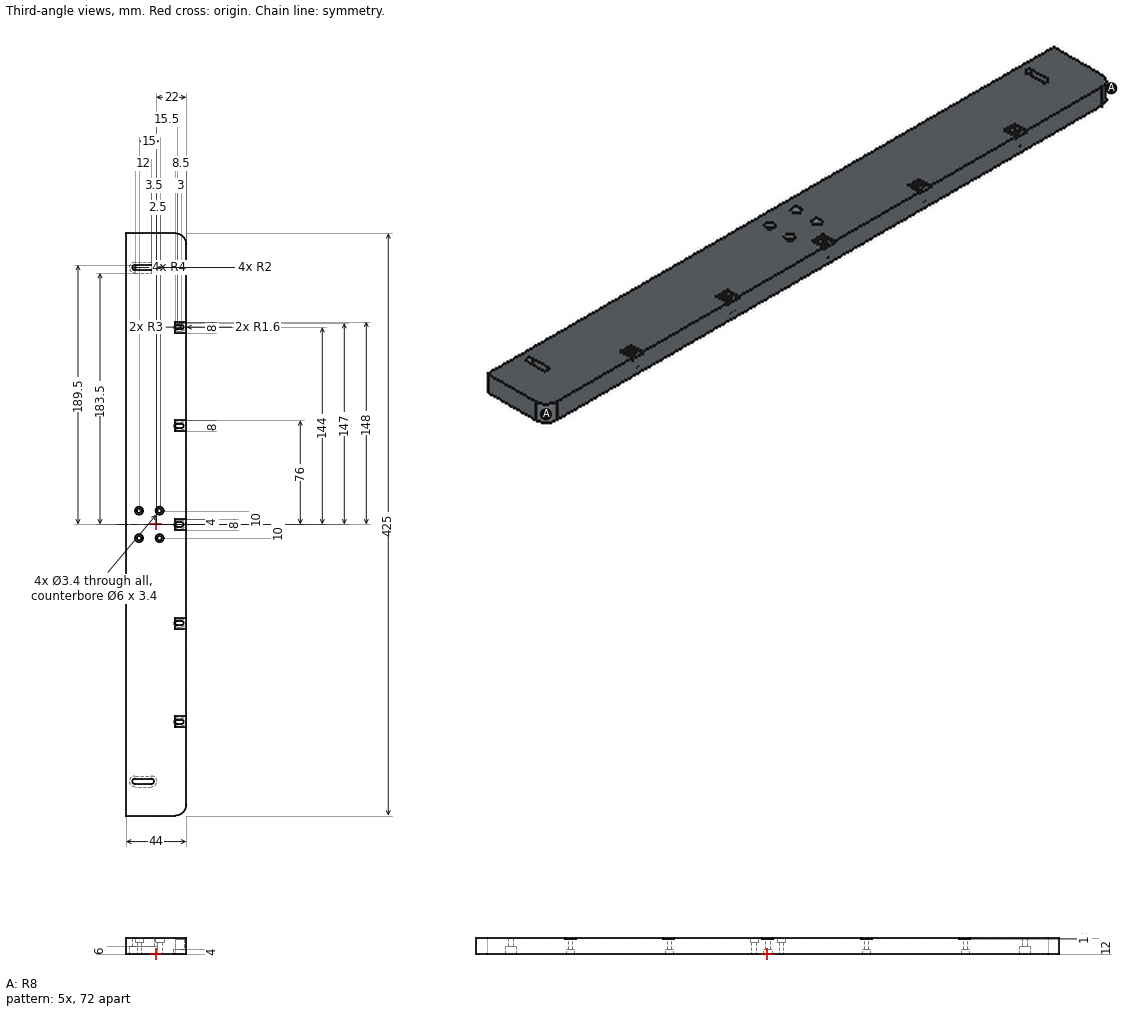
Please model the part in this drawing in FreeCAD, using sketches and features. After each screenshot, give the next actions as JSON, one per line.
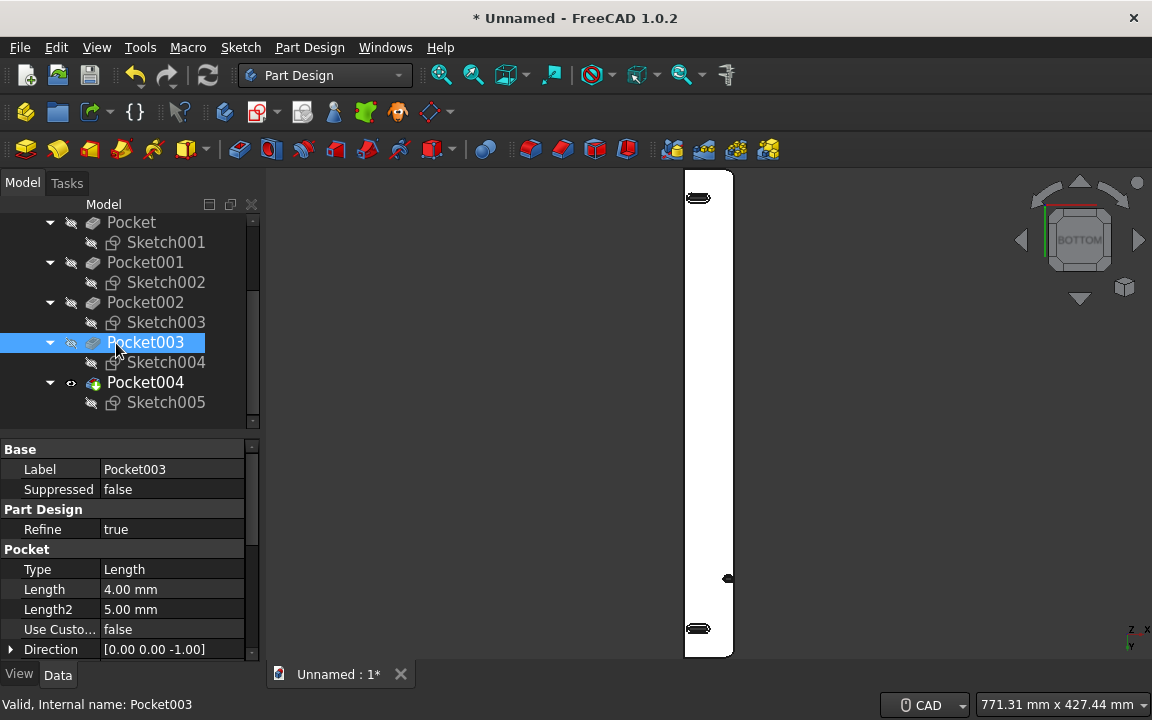
{"action": "left_click", "coordinate": [116, 383], "text": "ctrl"}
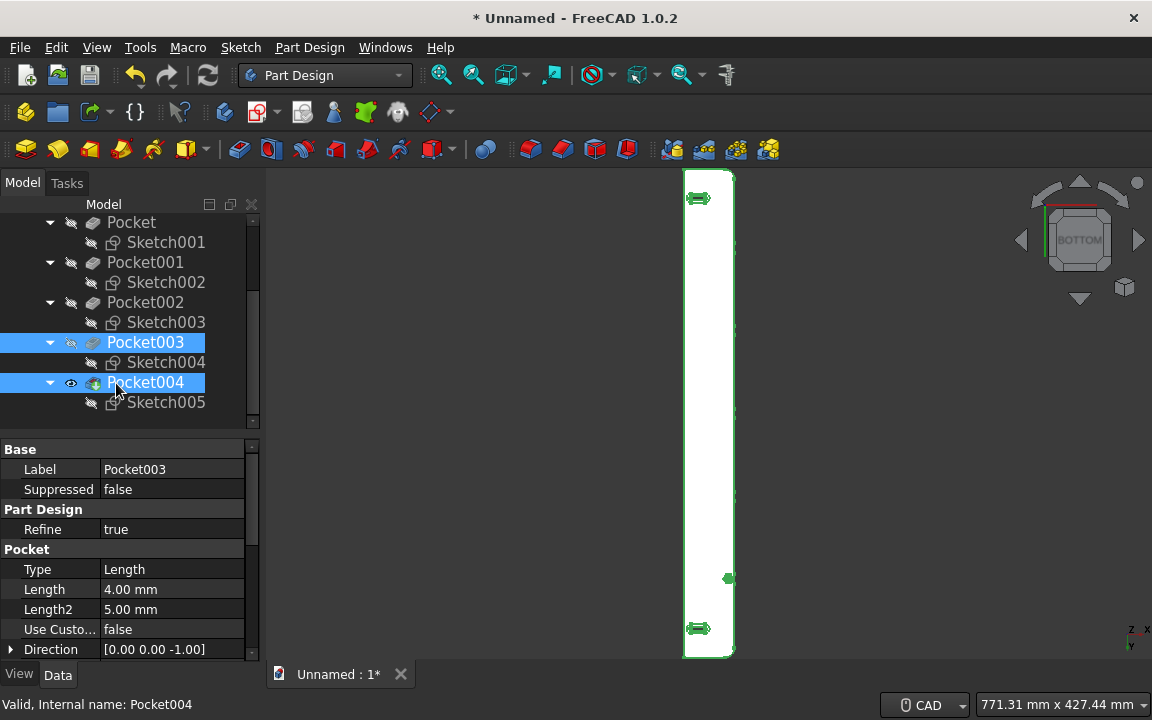
{"action": "left_click", "coordinate": [704, 150]}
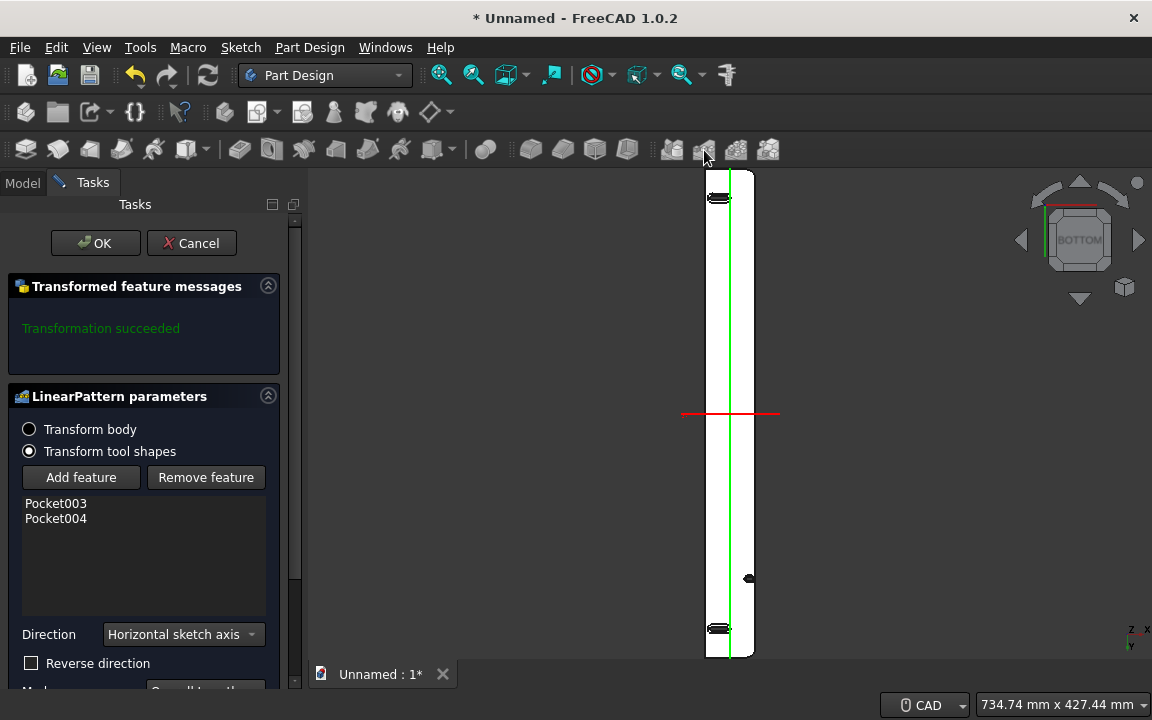
{"action": "left_click", "coordinate": [184, 634]}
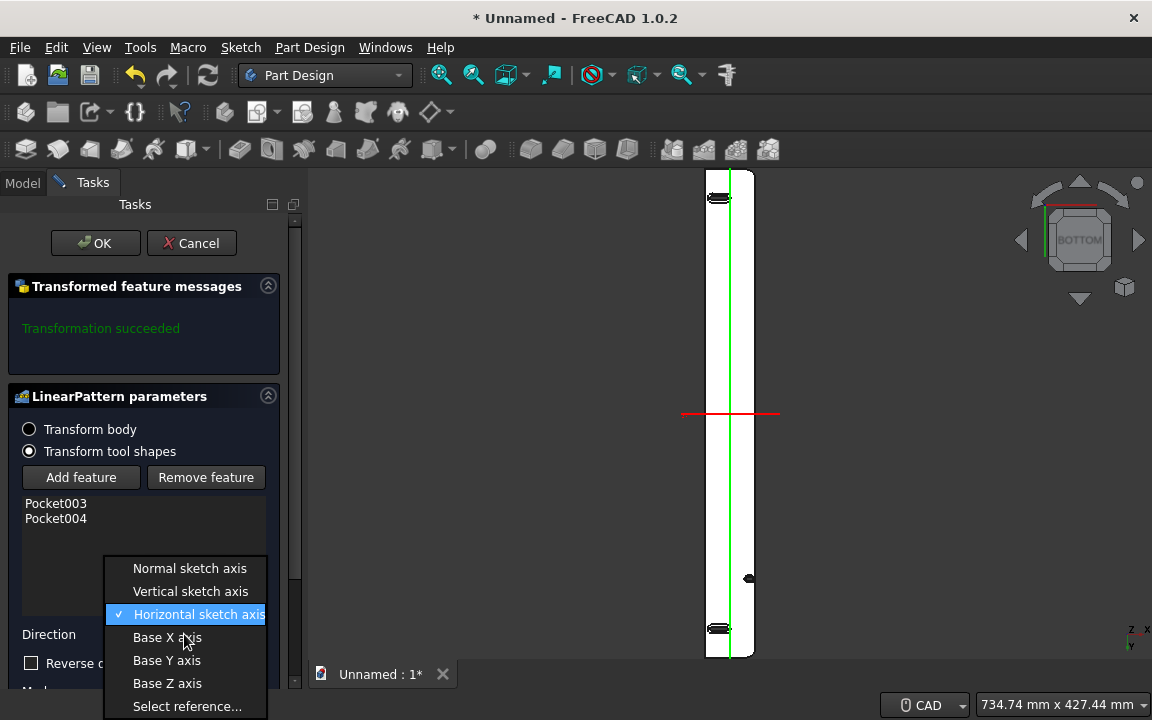
{"action": "left_click", "coordinate": [184, 660]}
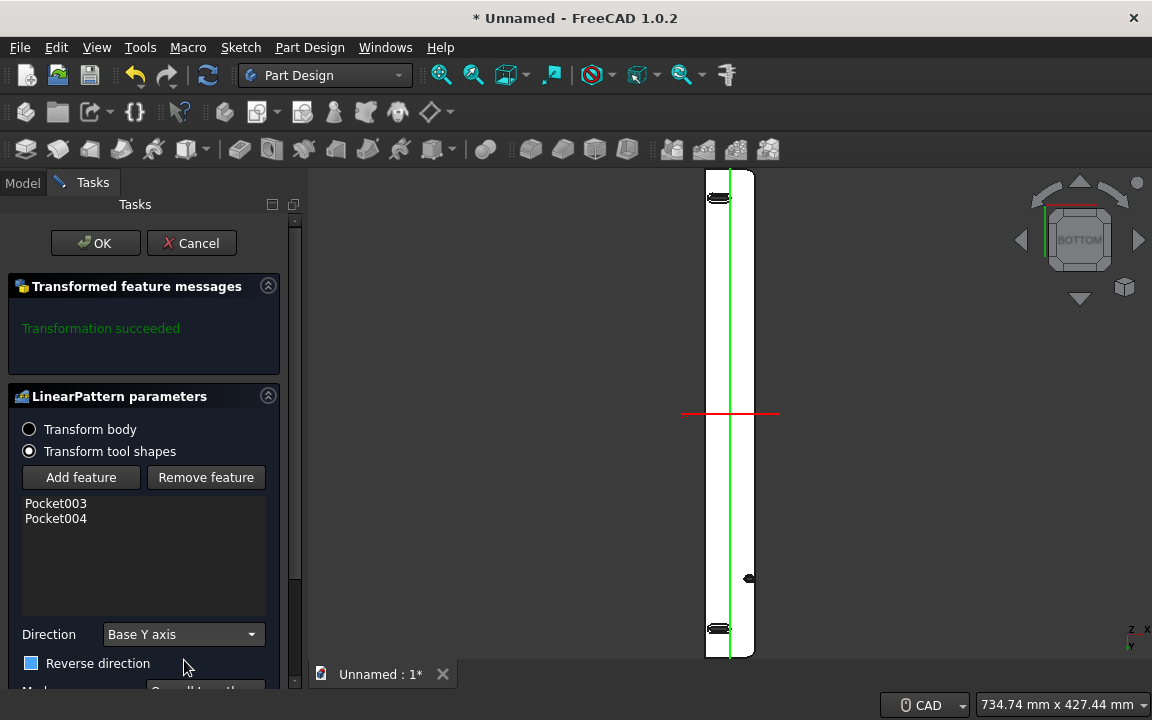
{"action": "scroll", "coordinate": [295, 451], "scroll_direction": "down", "scroll_amount": 2}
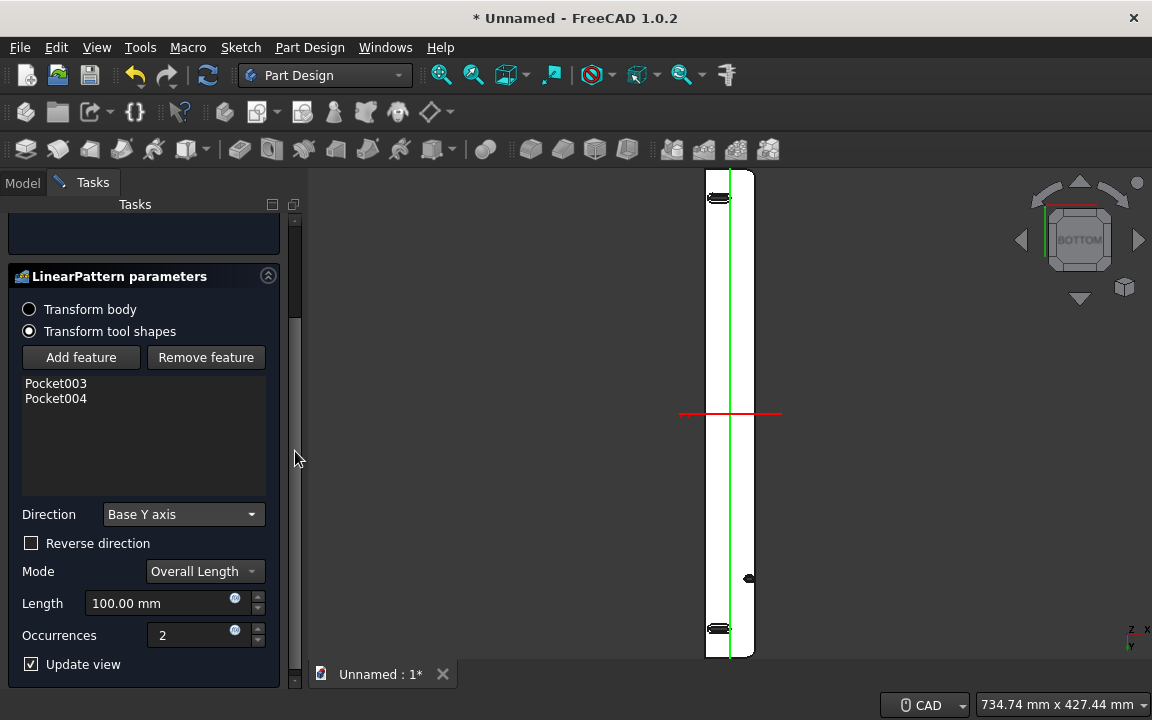
{"action": "left_click", "coordinate": [206, 572]}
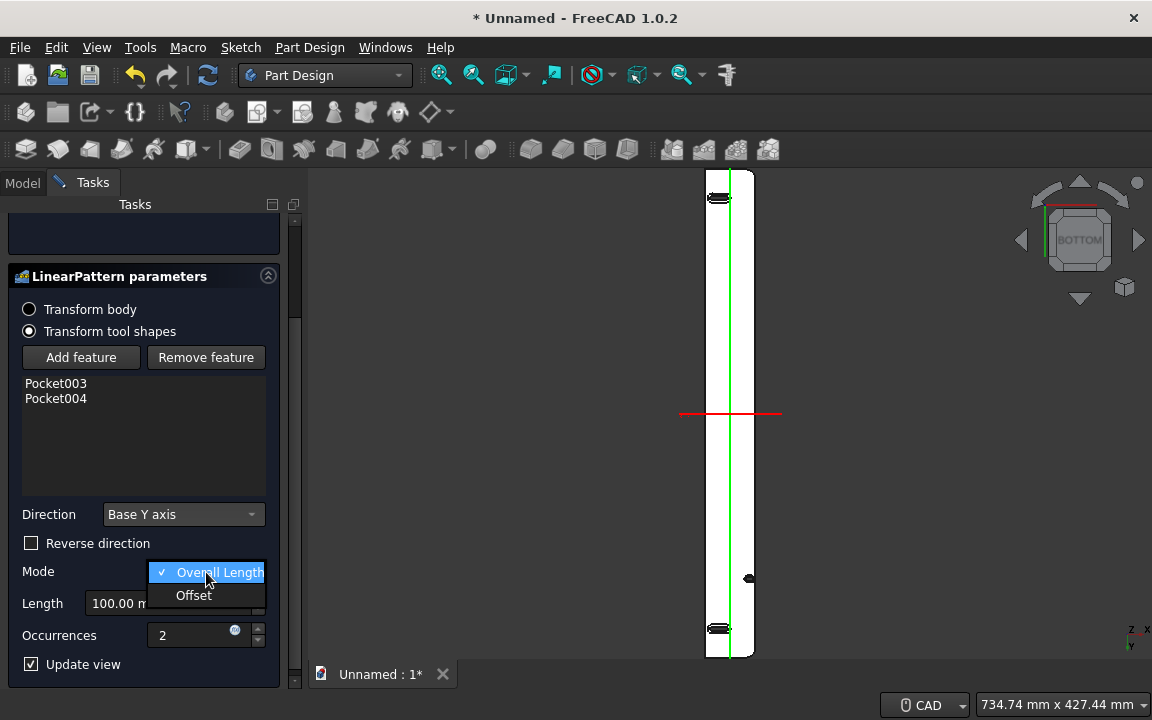
{"action": "left_click", "coordinate": [206, 596]}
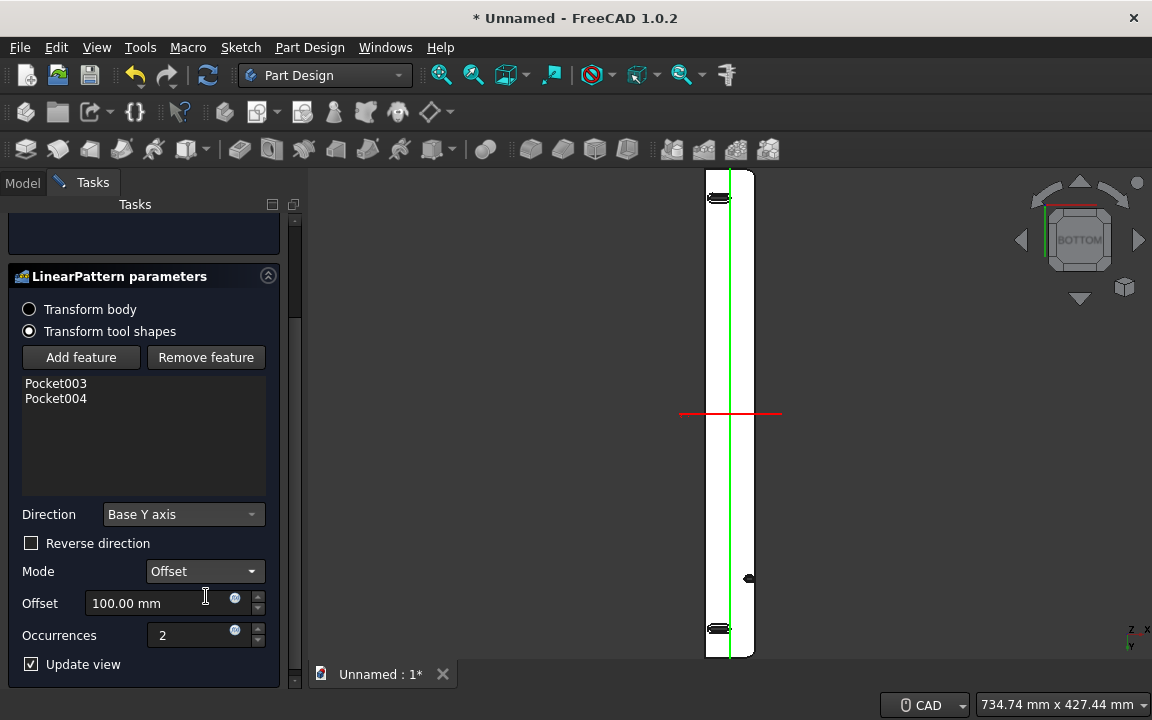
{"action": "triple_click", "coordinate": [168, 603]}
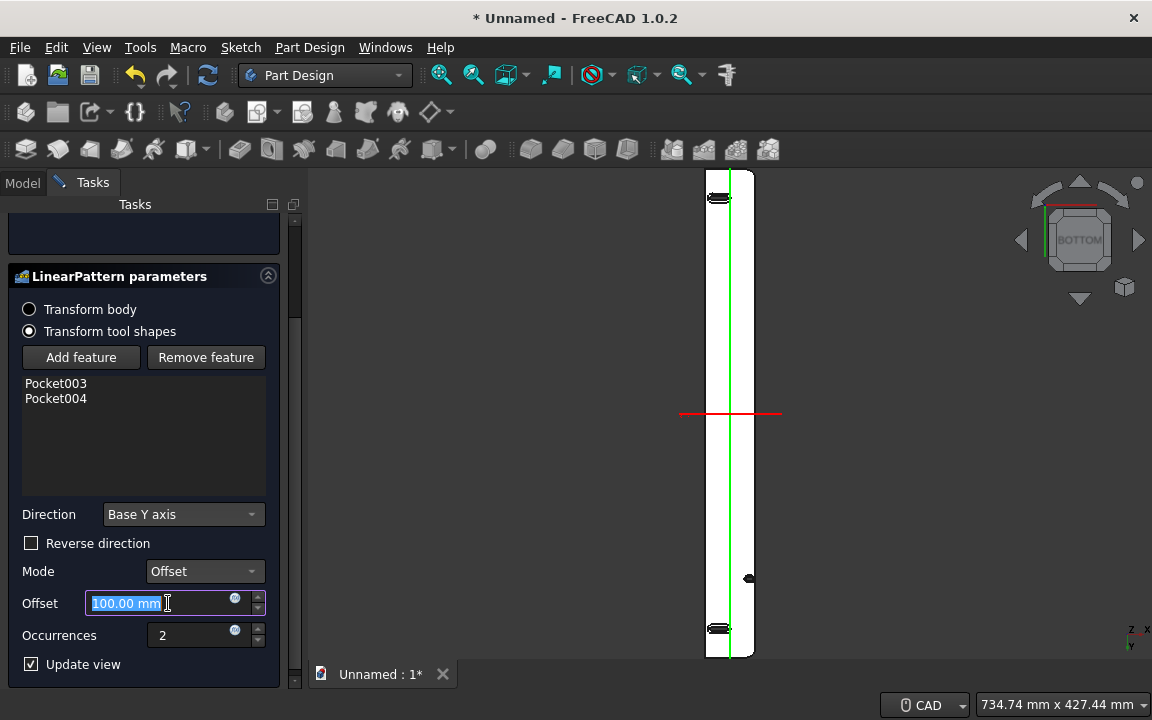
{"action": "type", "text": "72"}
{"action": "key", "text": "Tab"}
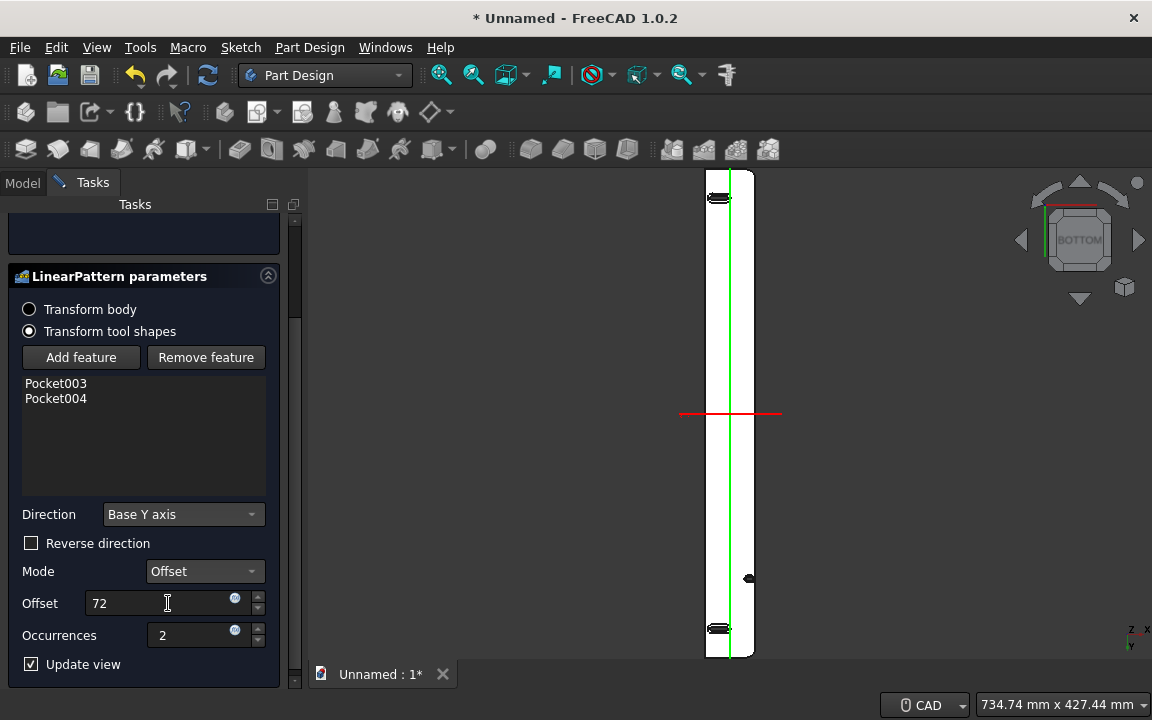
{"action": "triple_click", "coordinate": [198, 635]}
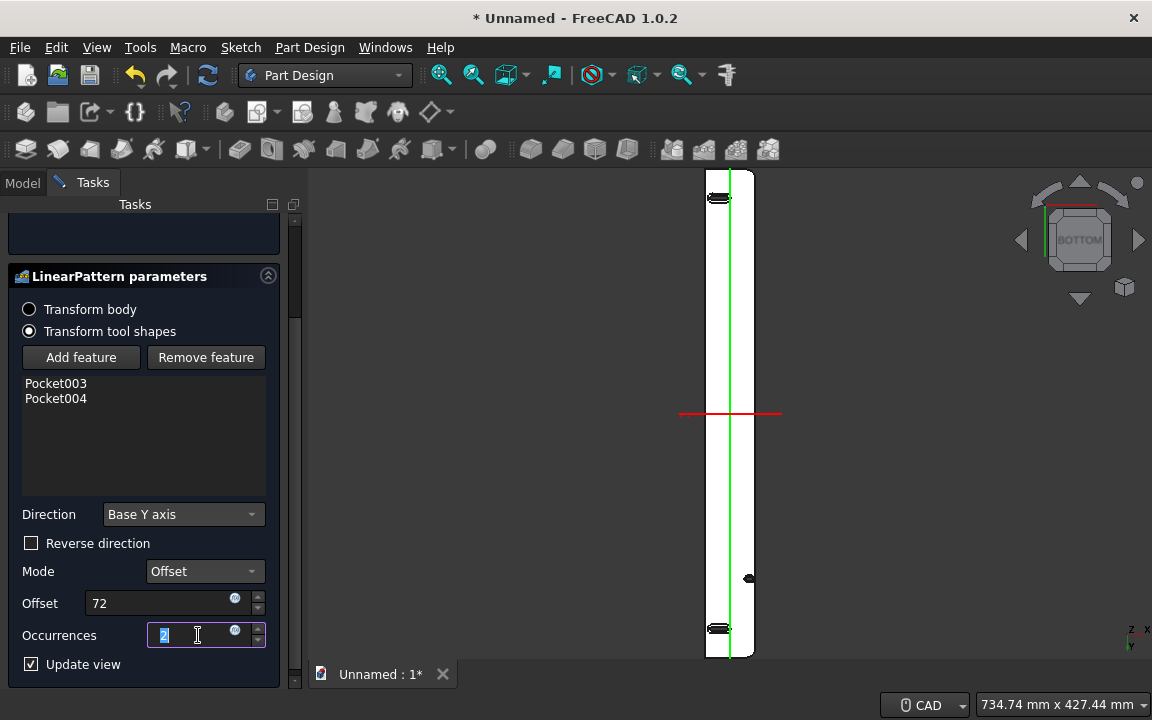
{"action": "type", "text": "5"}
{"action": "key", "text": "Tab"}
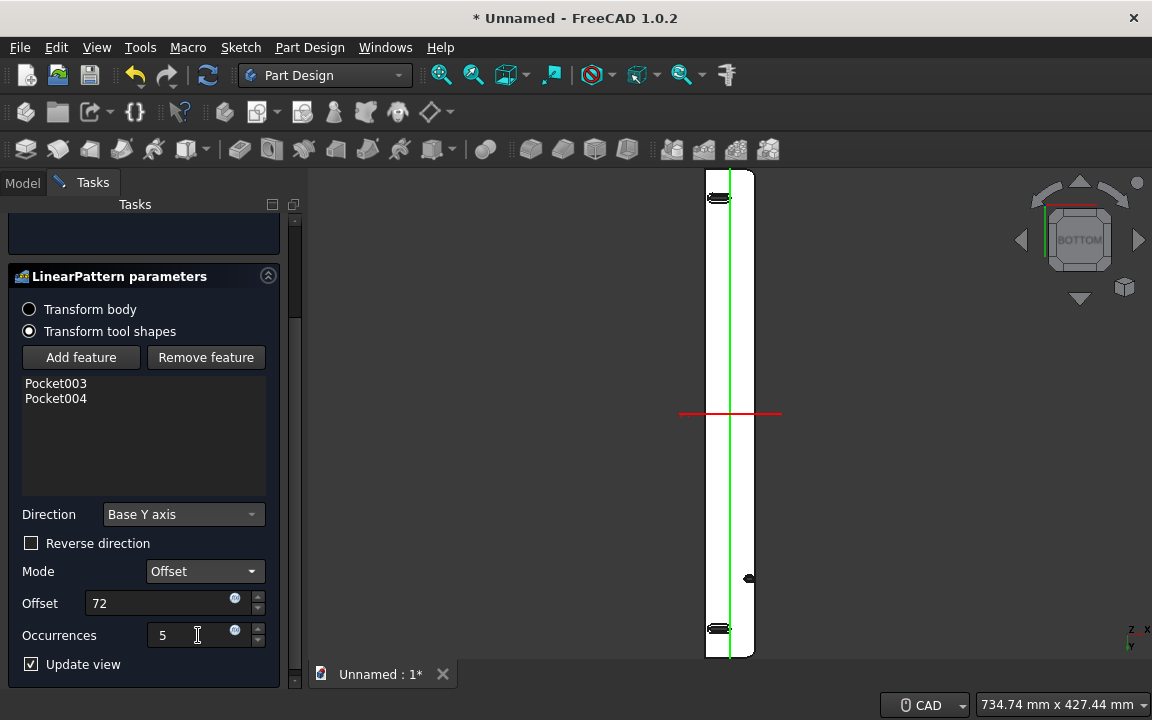
{"action": "left_click", "coordinate": [30, 543]}